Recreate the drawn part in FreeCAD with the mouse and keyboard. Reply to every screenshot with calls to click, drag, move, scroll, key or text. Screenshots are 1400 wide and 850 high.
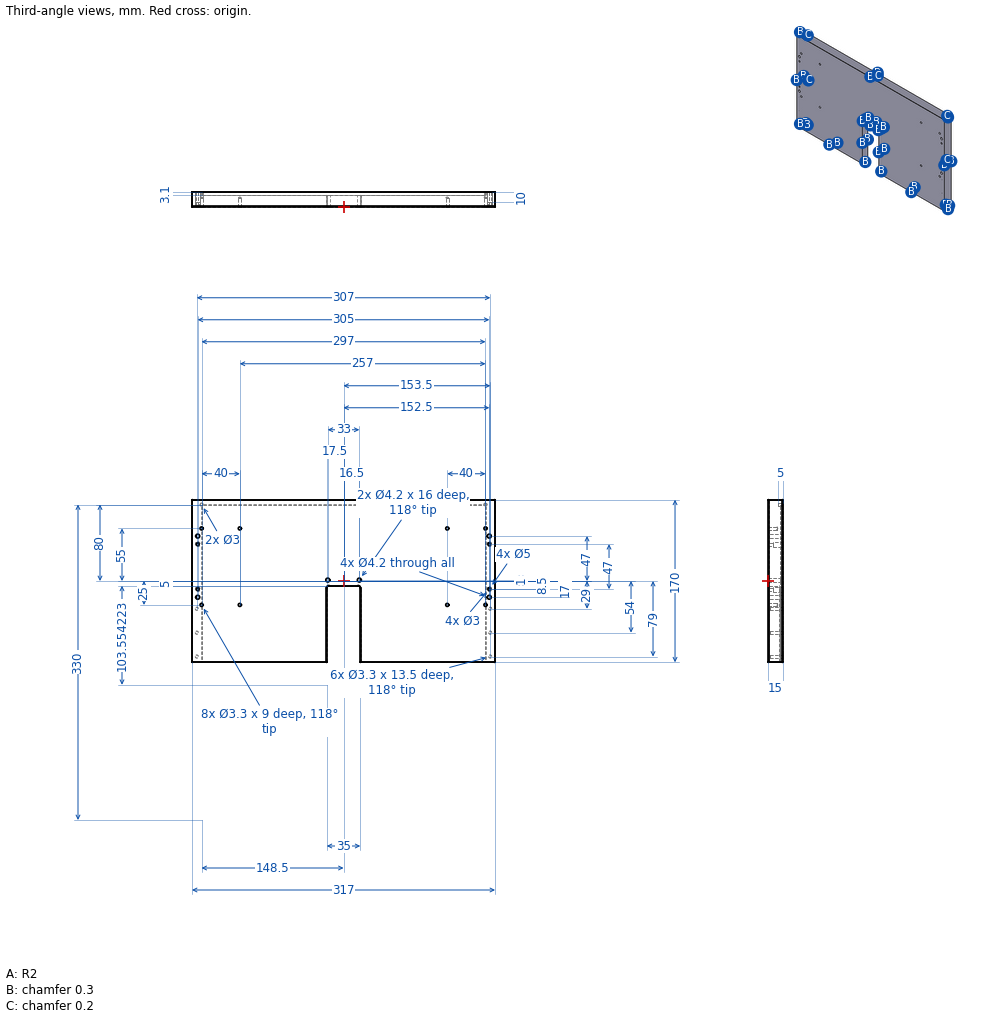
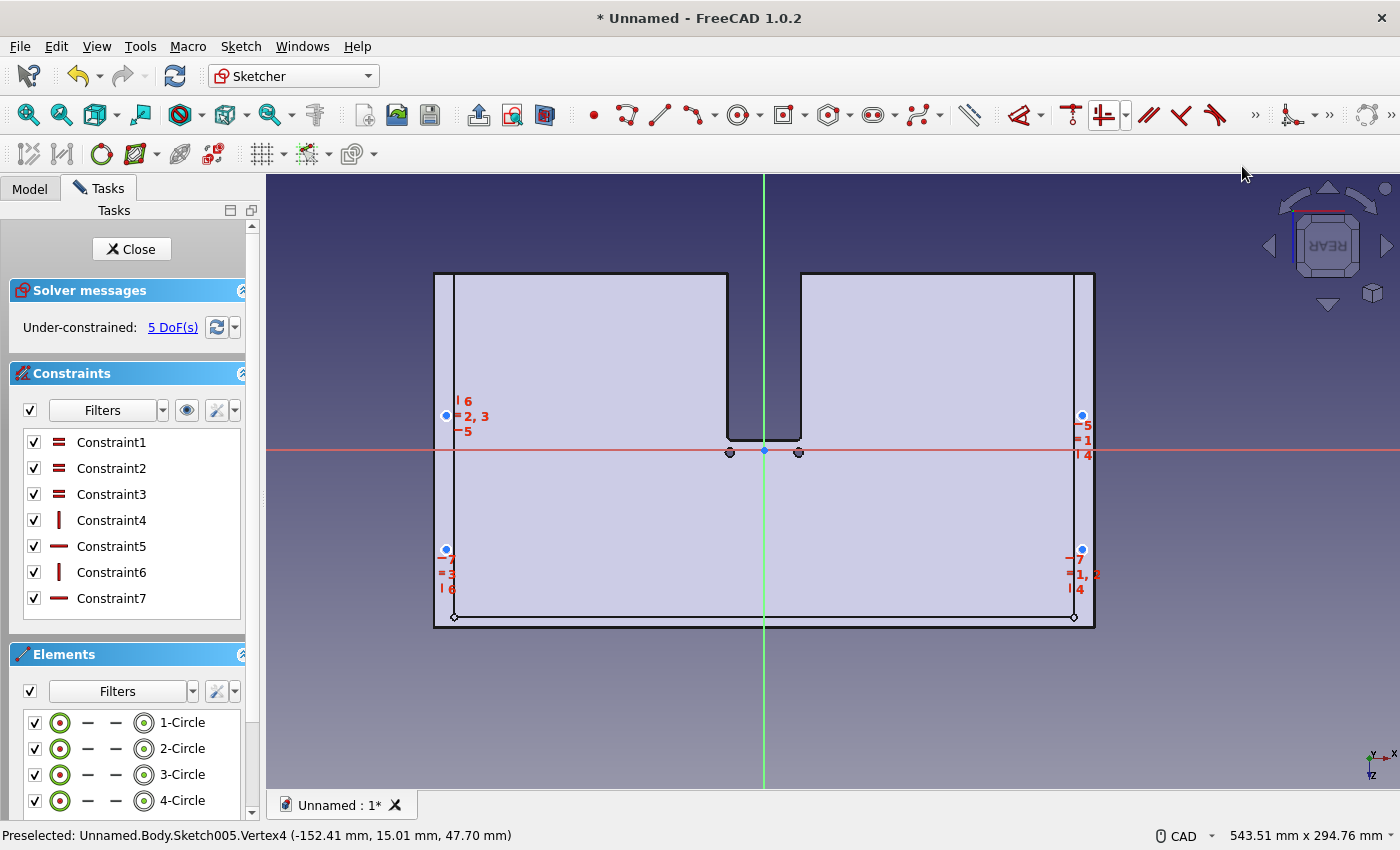
click(1018, 116)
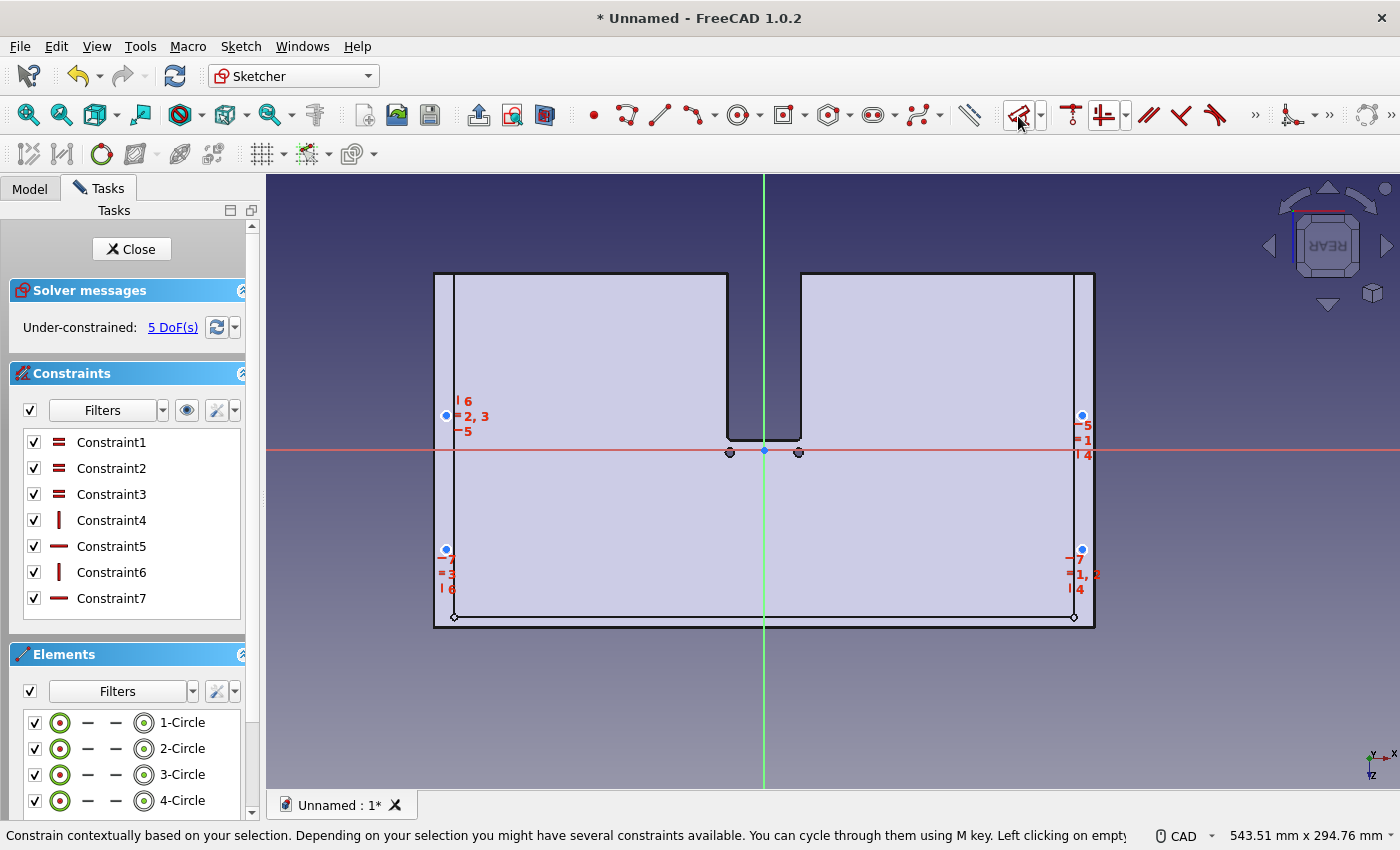
scroll(1086, 412, up, 8)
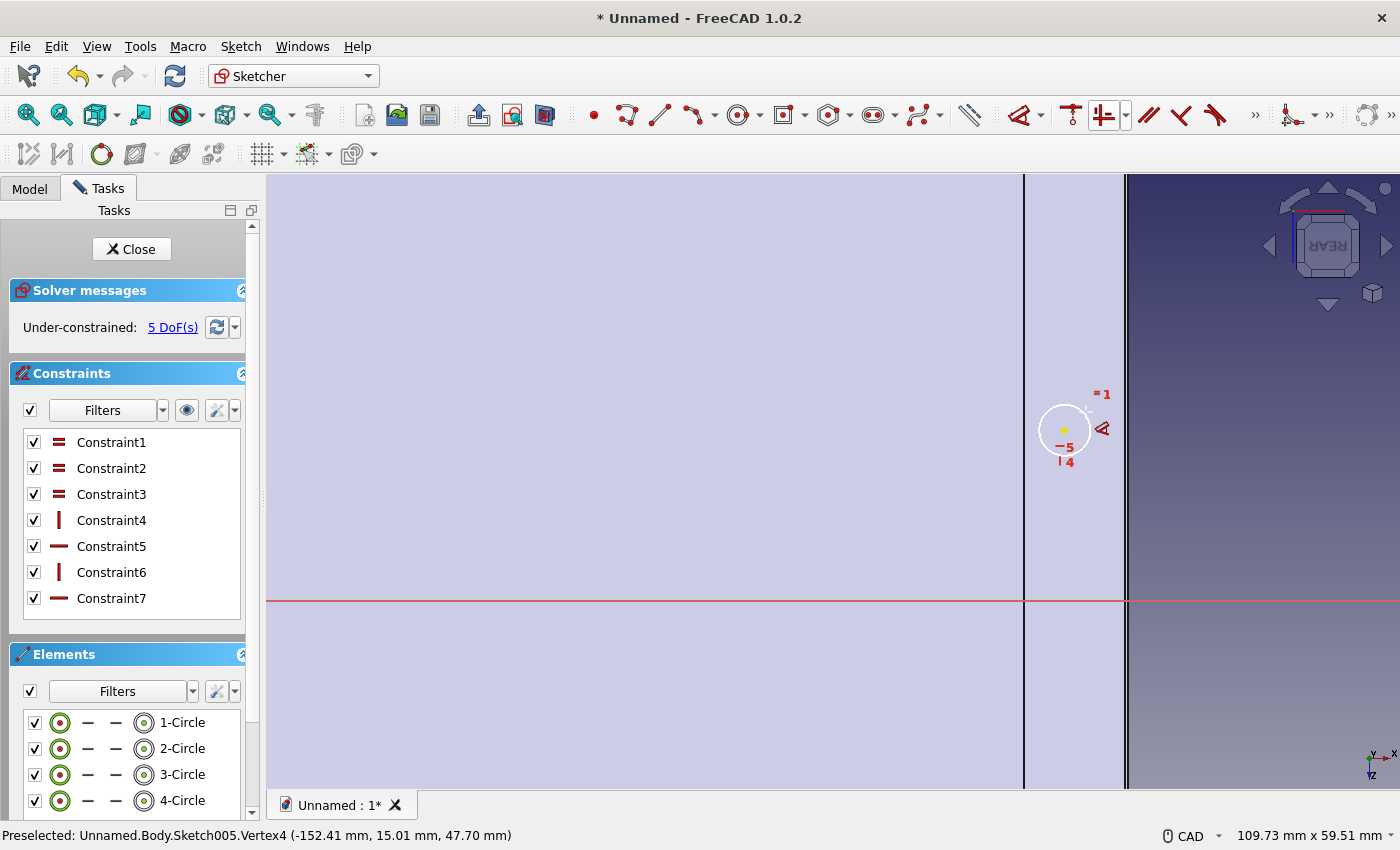
click(1083, 412)
click(1106, 389)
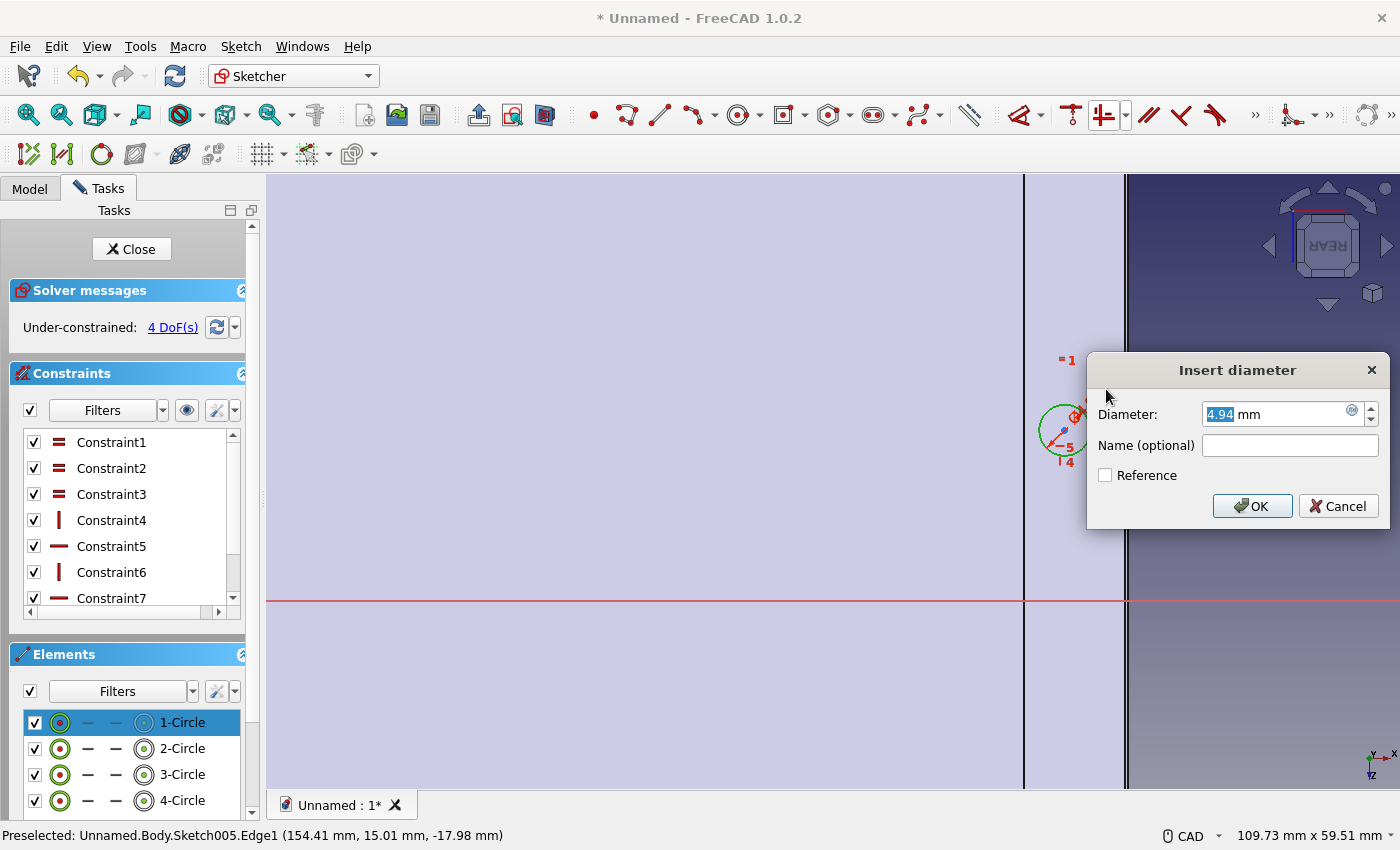
text(4.2)
key(Return)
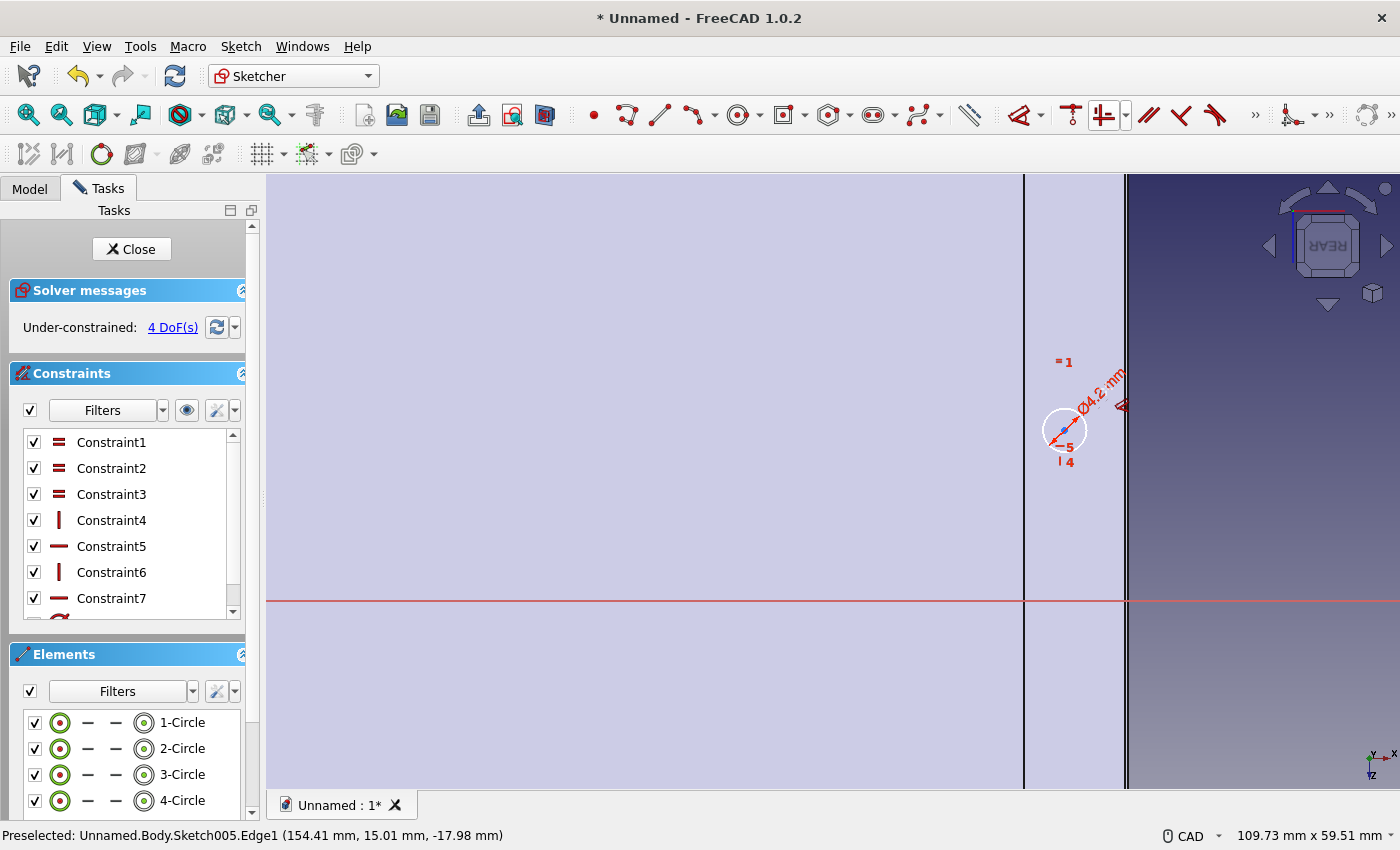
scroll(1087, 412, down, 8)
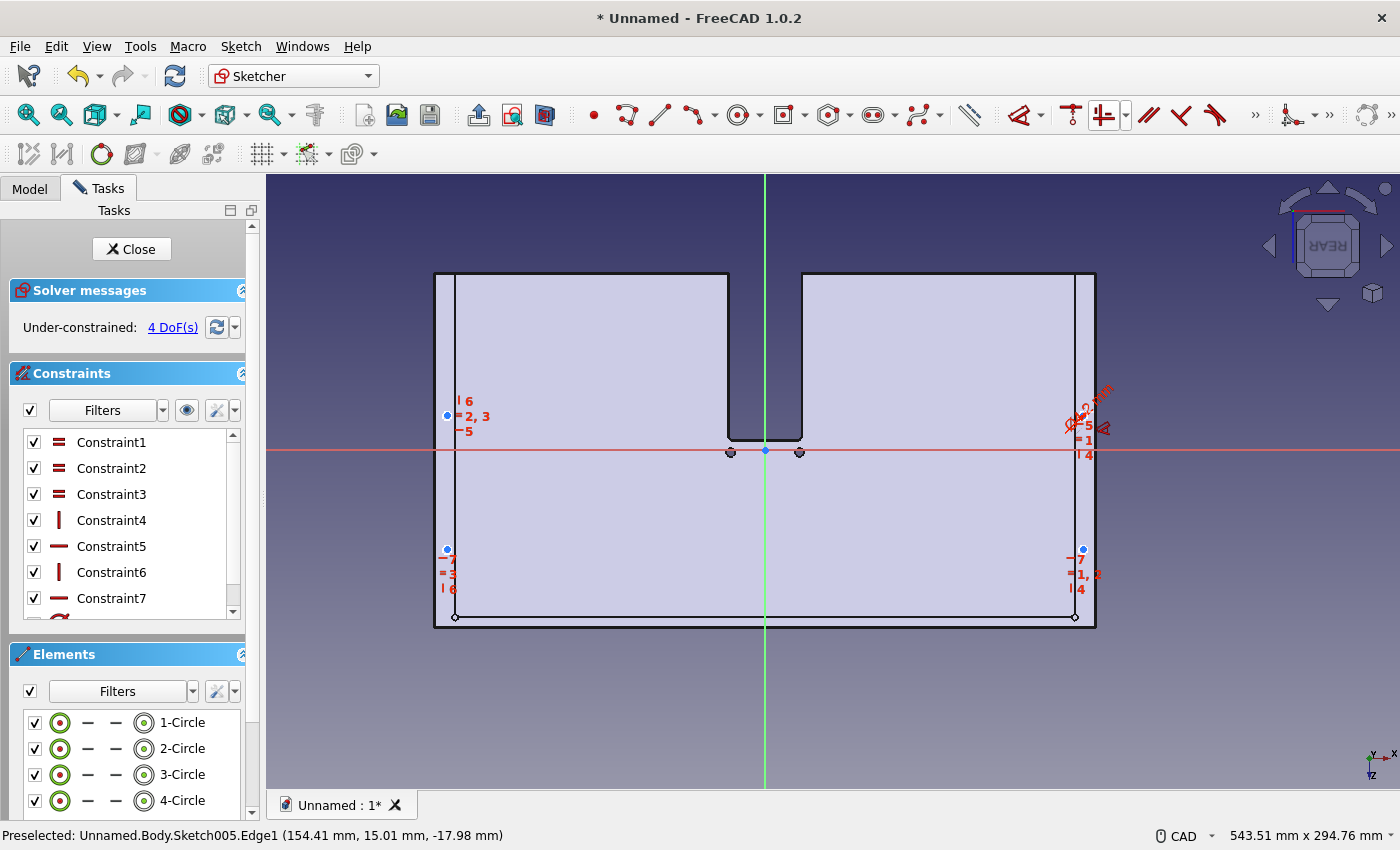
click(1083, 416)
click(1117, 433)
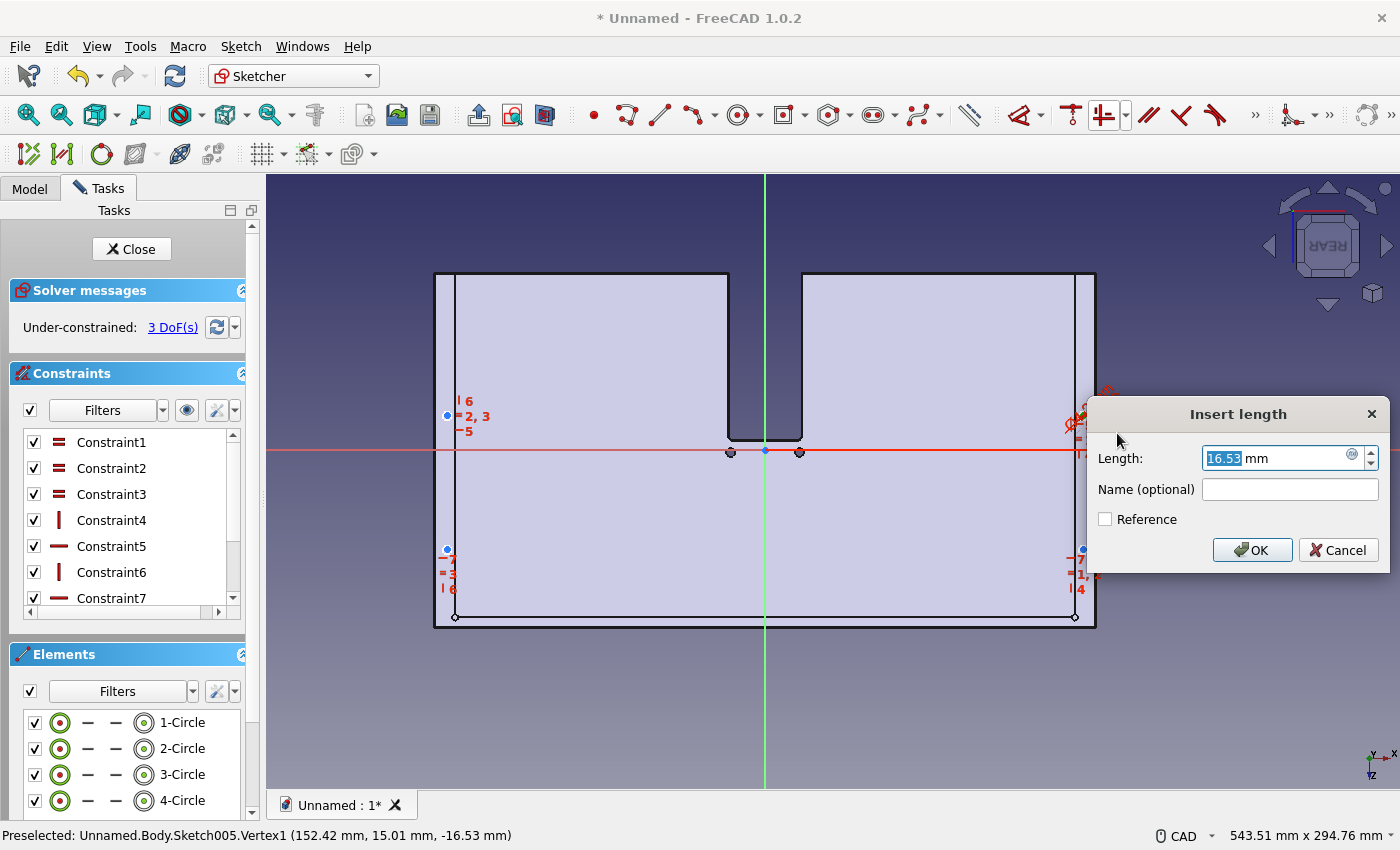
text(17)
key(Return)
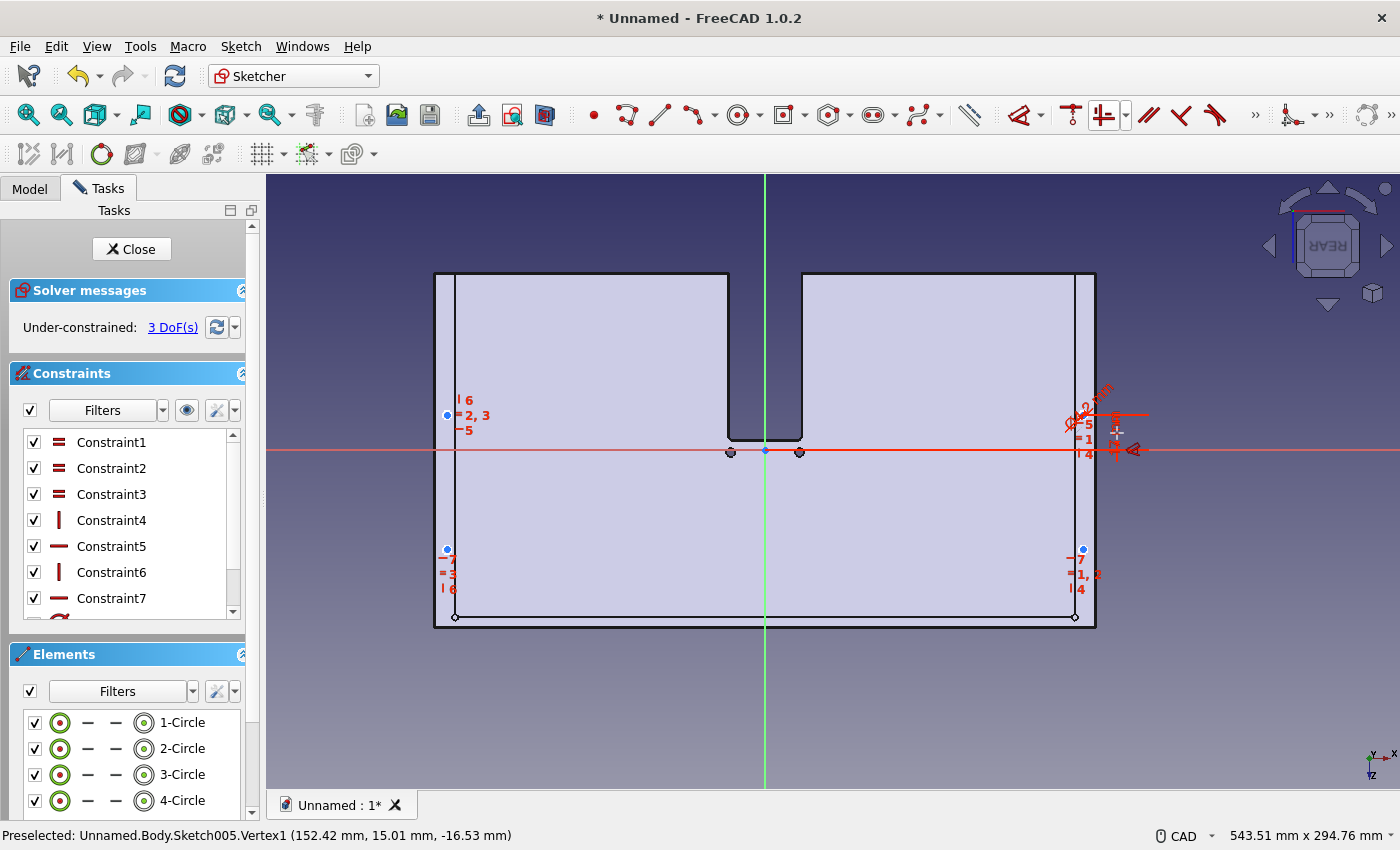
click(1083, 550)
click(1117, 500)